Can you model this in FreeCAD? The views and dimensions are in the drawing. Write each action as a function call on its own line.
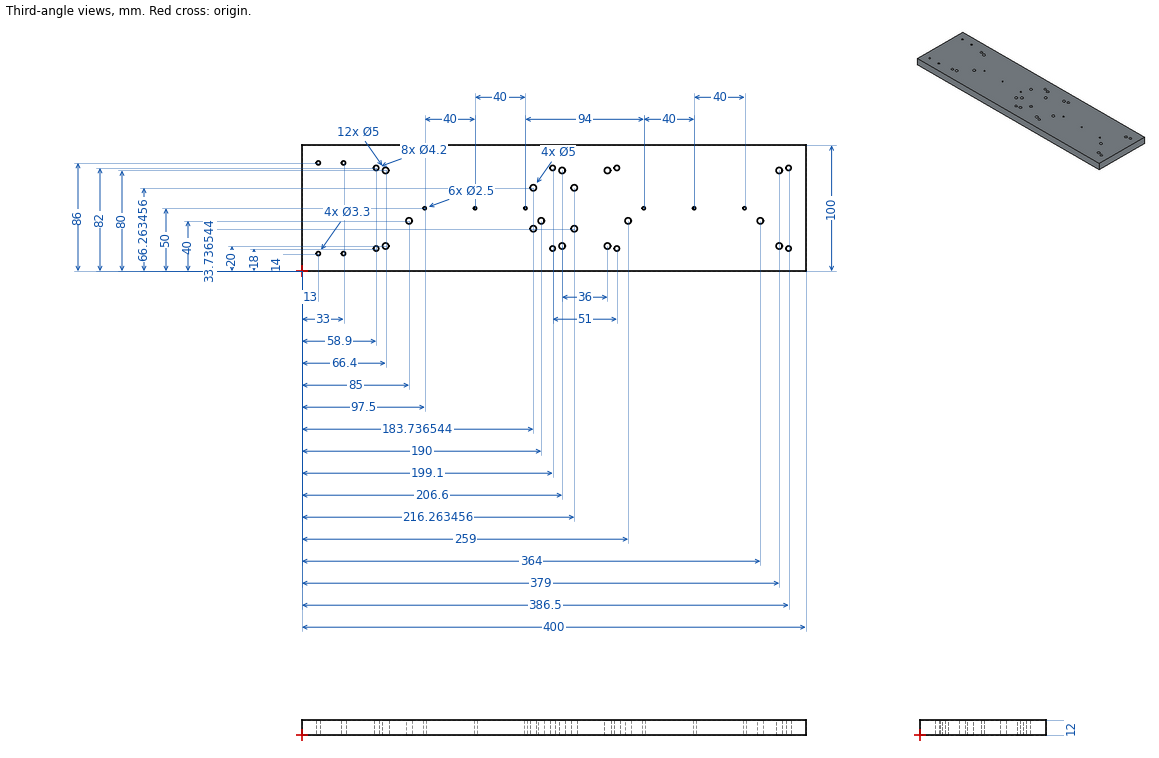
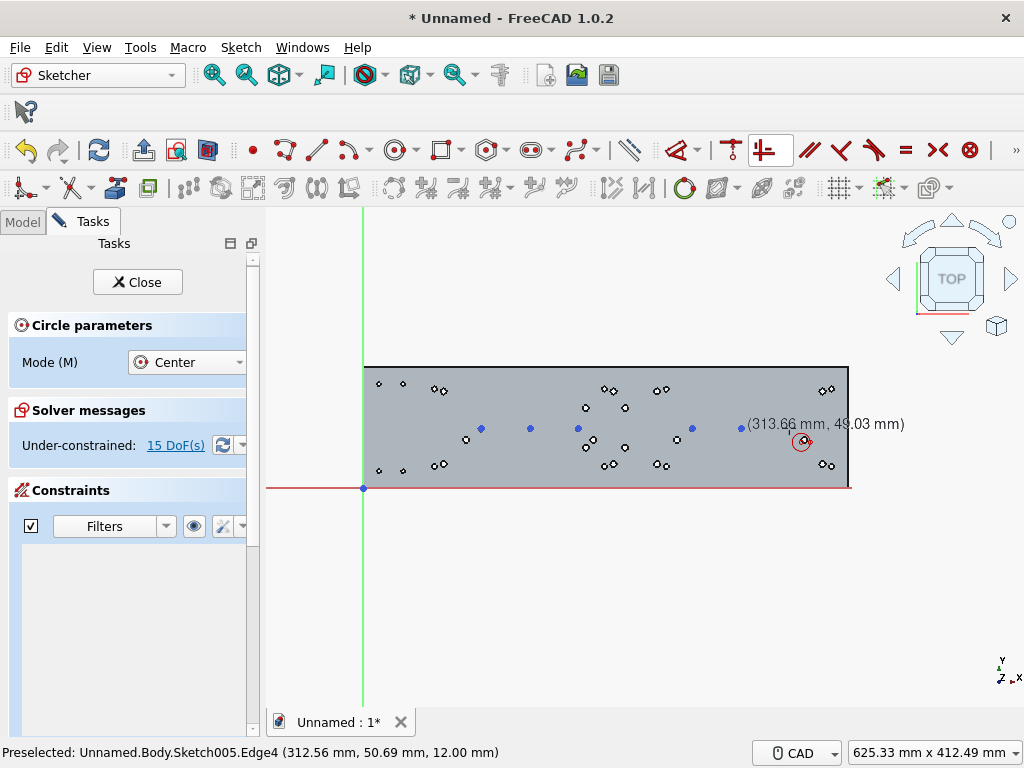
click(789, 428)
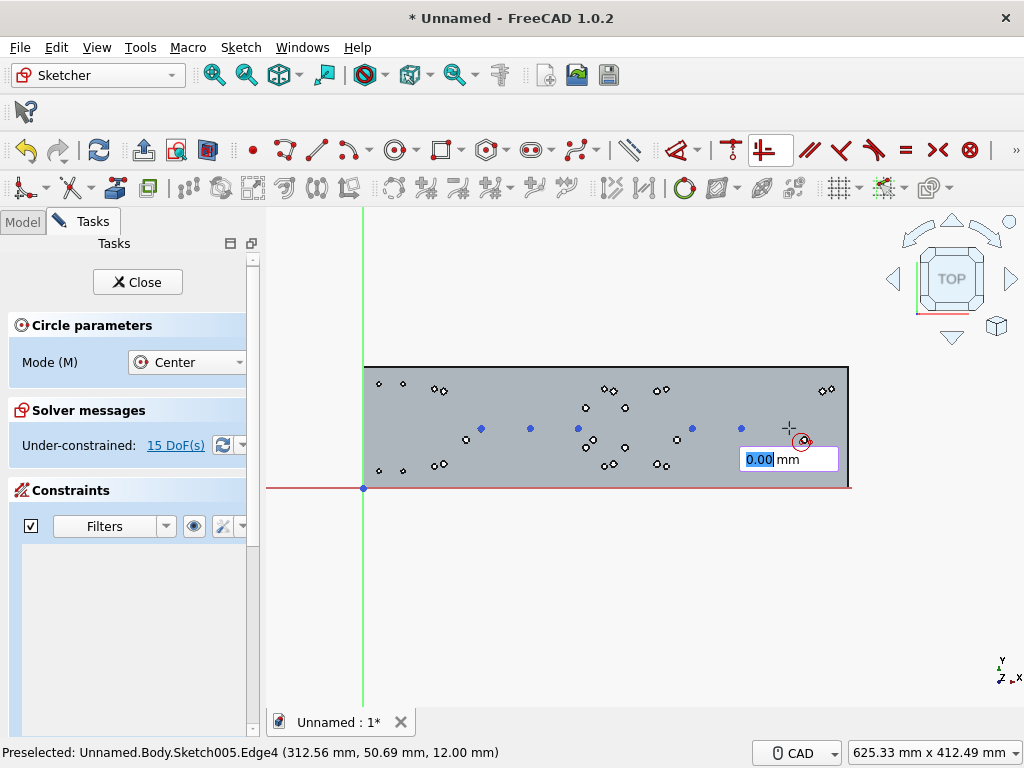
scroll(790, 427, up, 12)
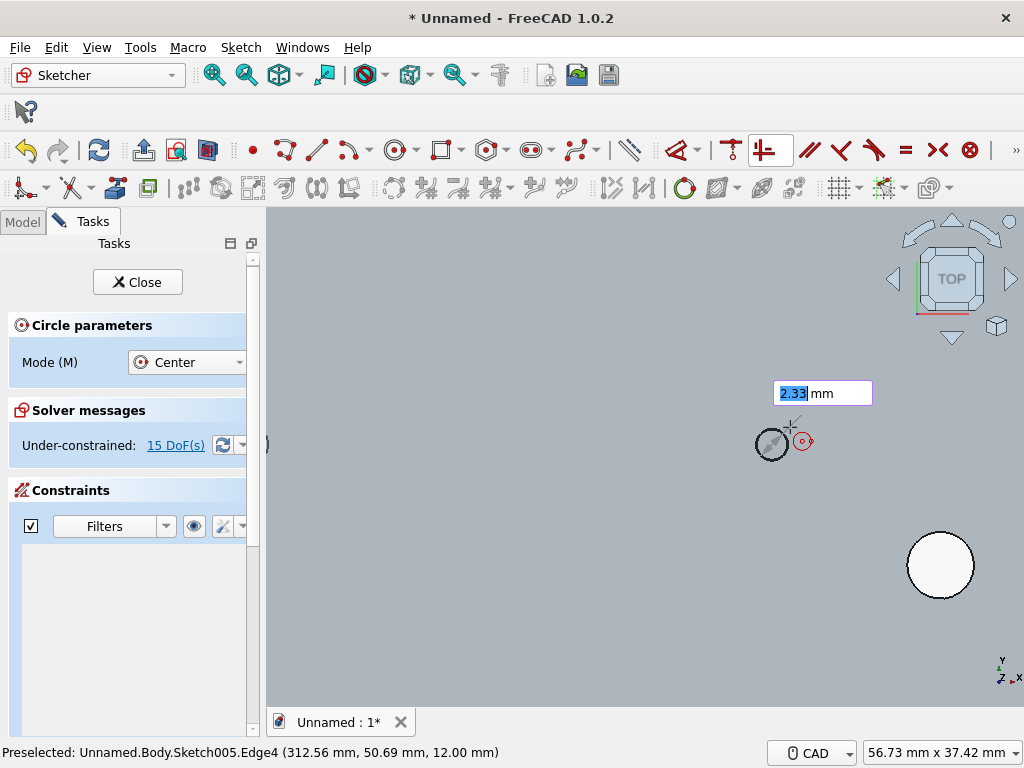
click(785, 420)
key(Escape)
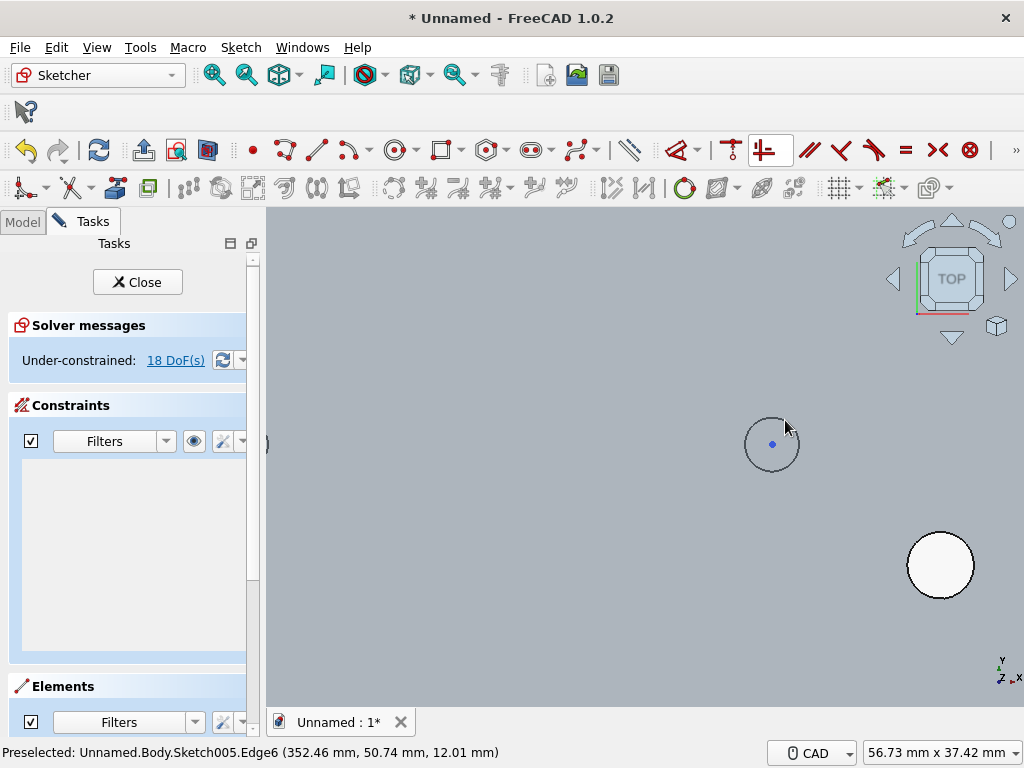
scroll(790, 427, down, 12)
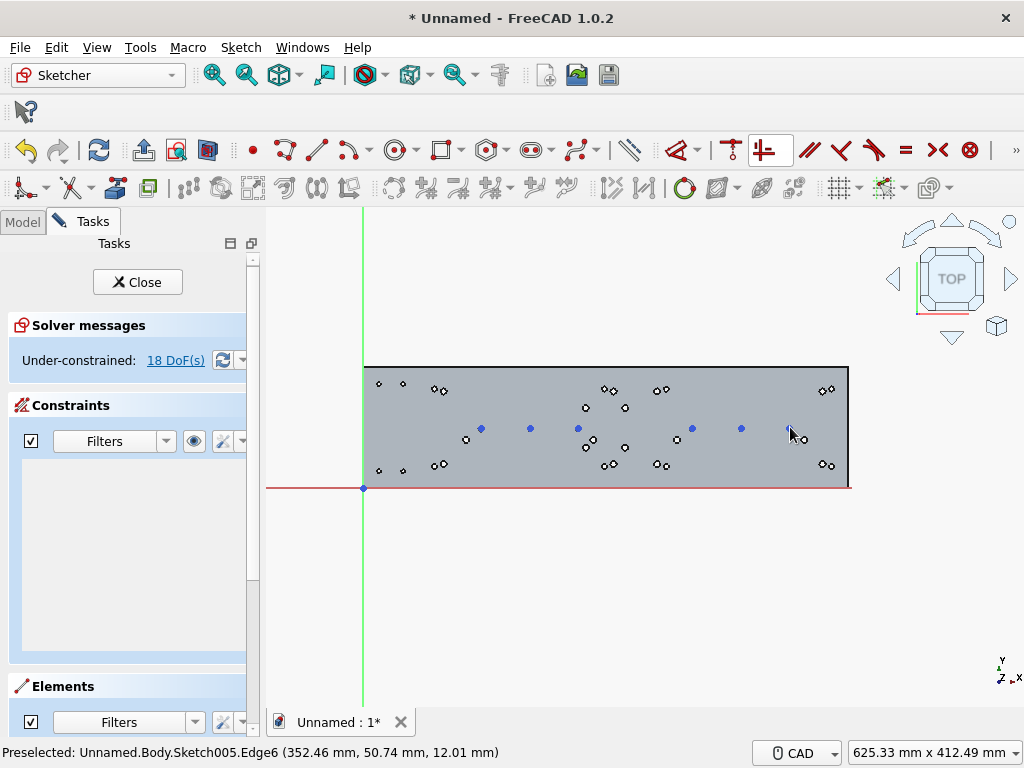
scroll(483, 427, up, 9)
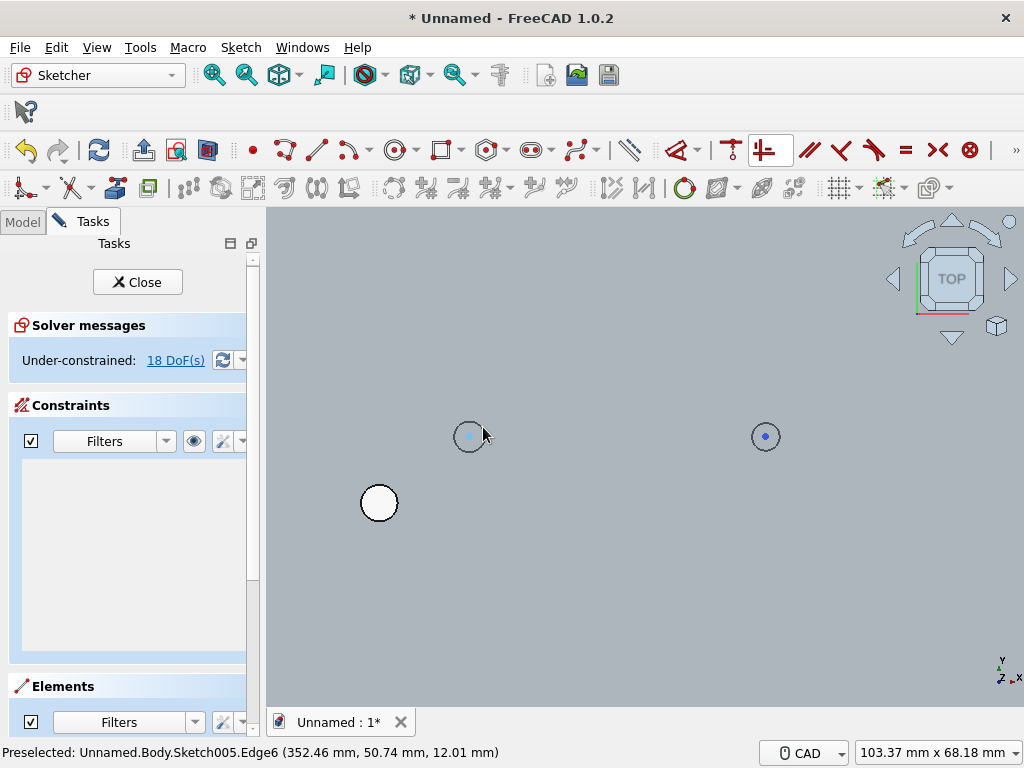
click(480, 426)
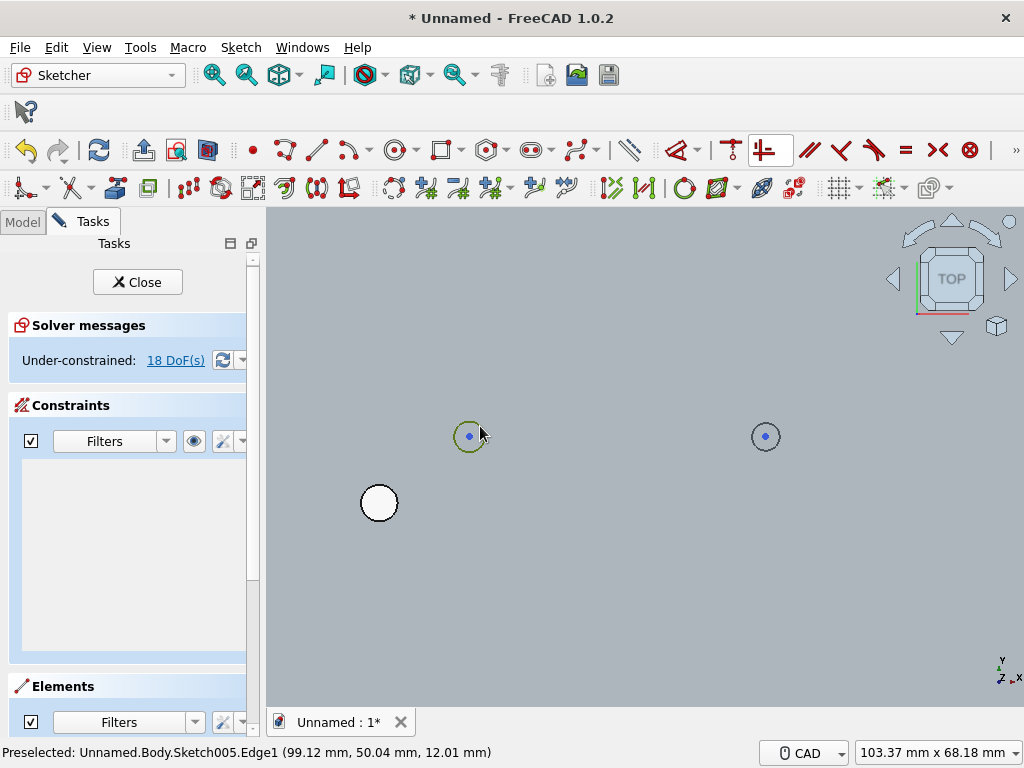
click(776, 427)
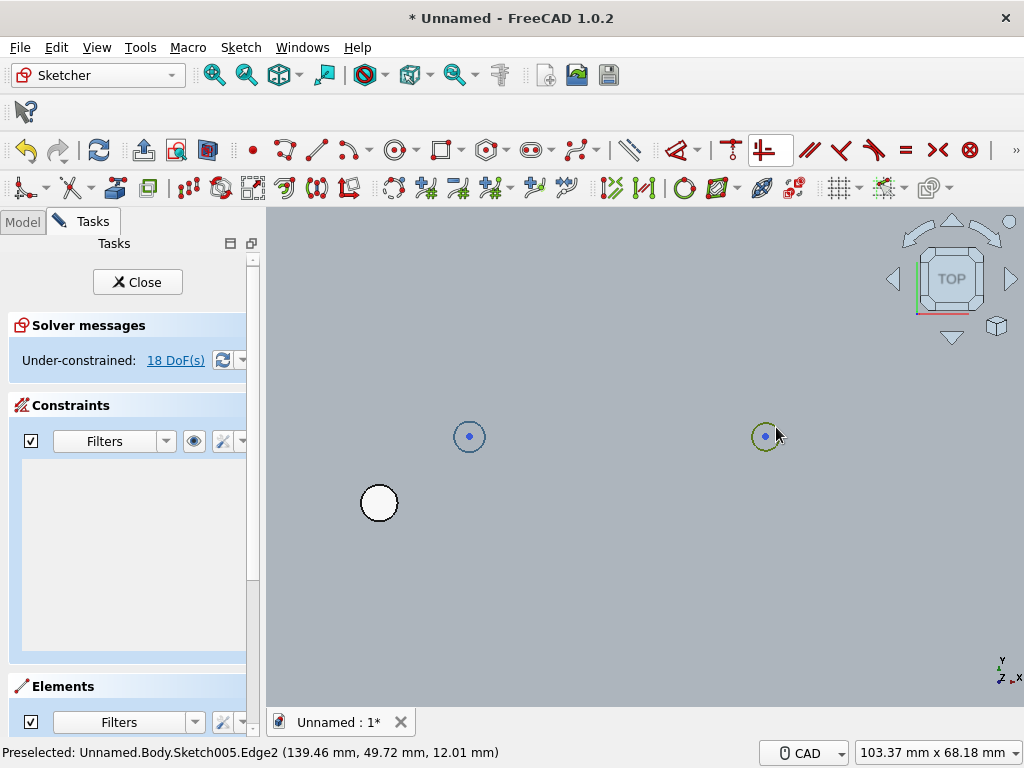
scroll(483, 427, down, 9)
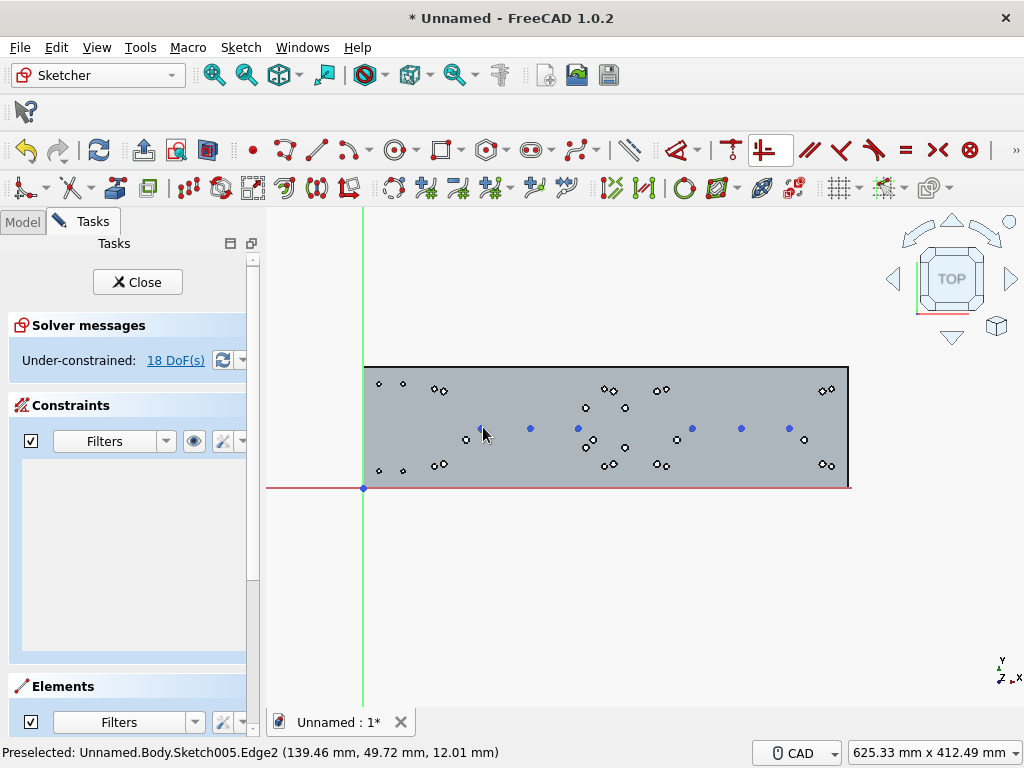
scroll(580, 427, up, 9)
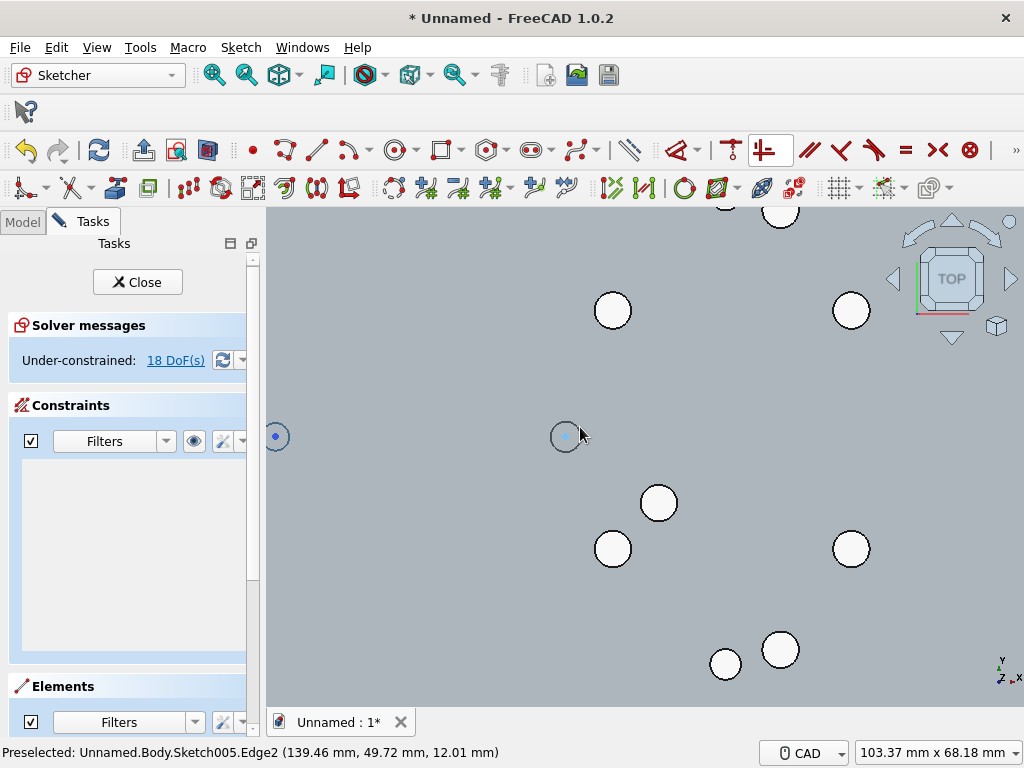
click(576, 426)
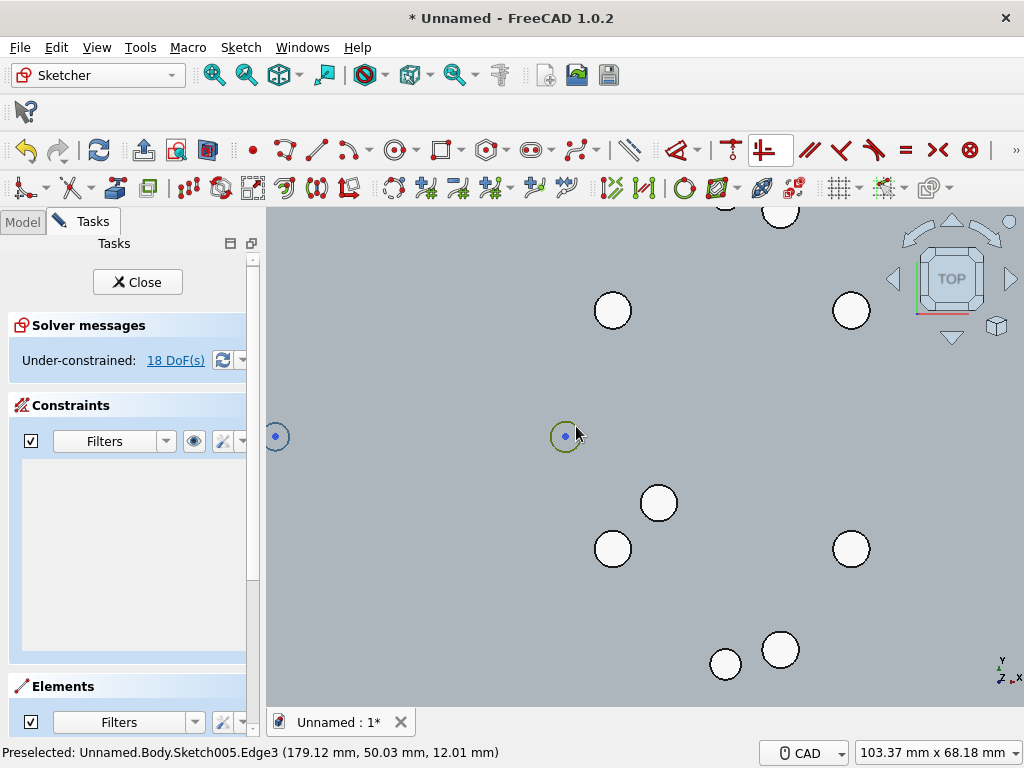
scroll(580, 427, down, 9)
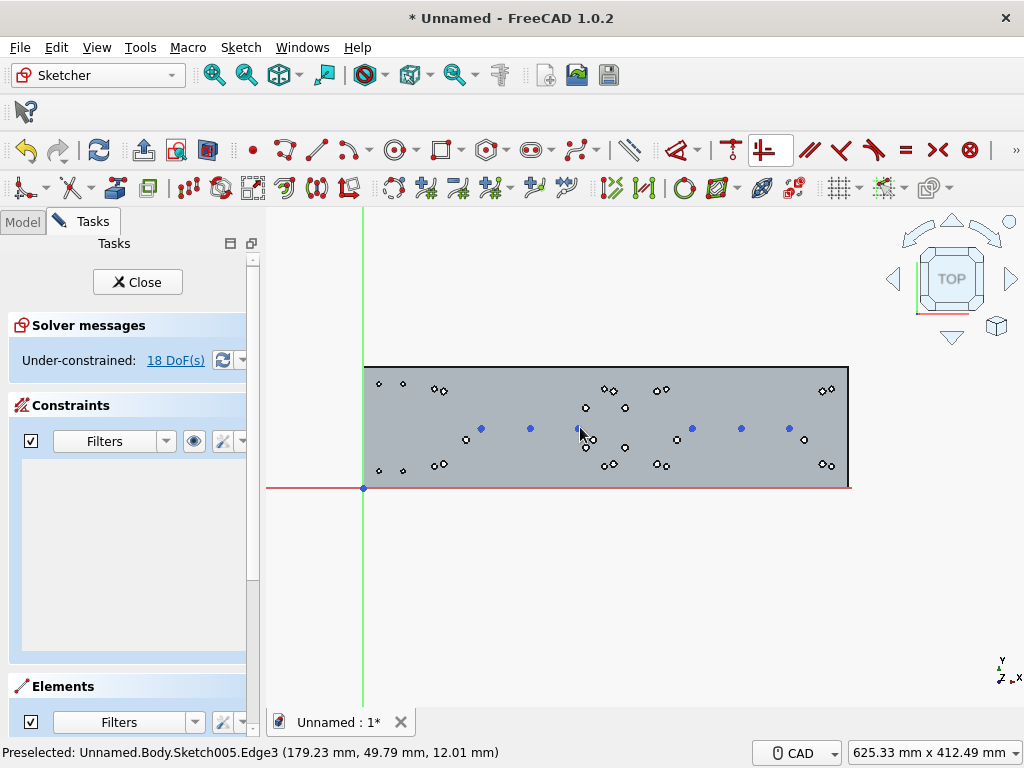
scroll(694, 427, up, 9)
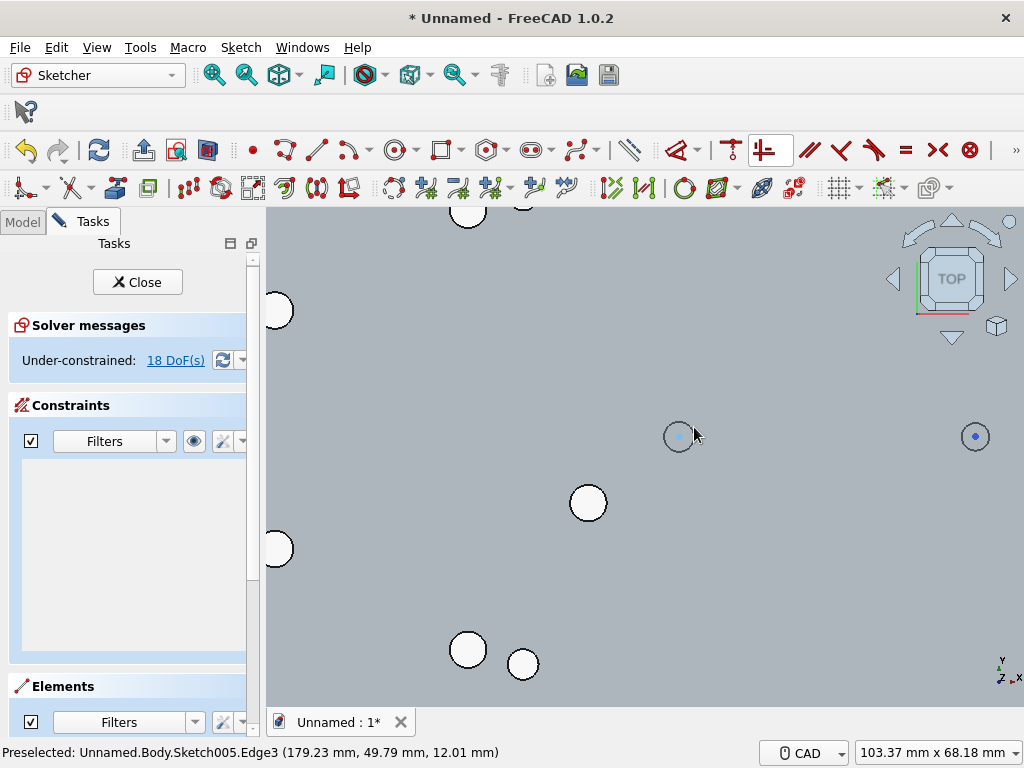
click(690, 426)